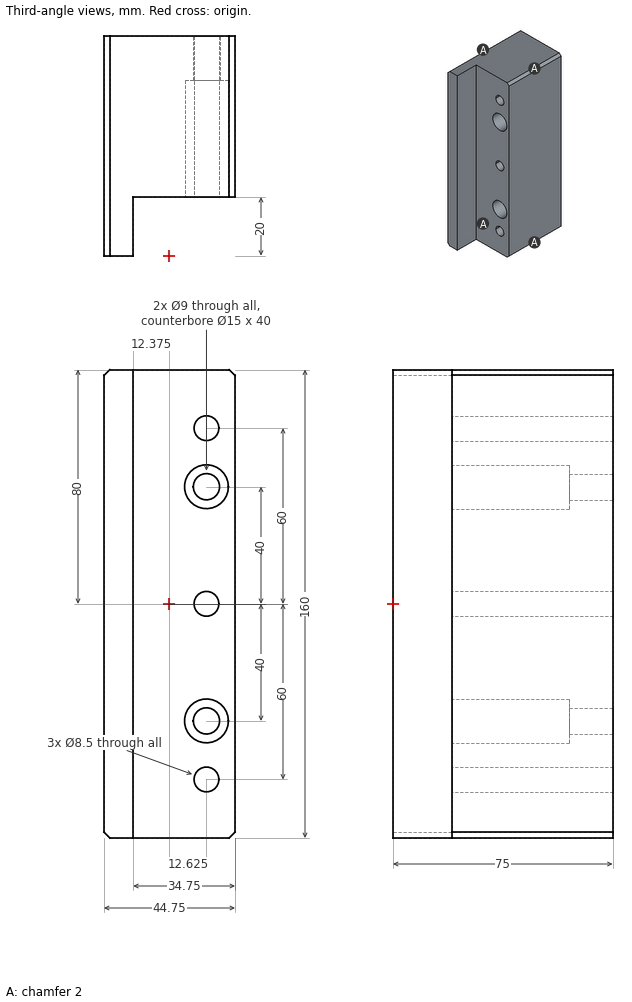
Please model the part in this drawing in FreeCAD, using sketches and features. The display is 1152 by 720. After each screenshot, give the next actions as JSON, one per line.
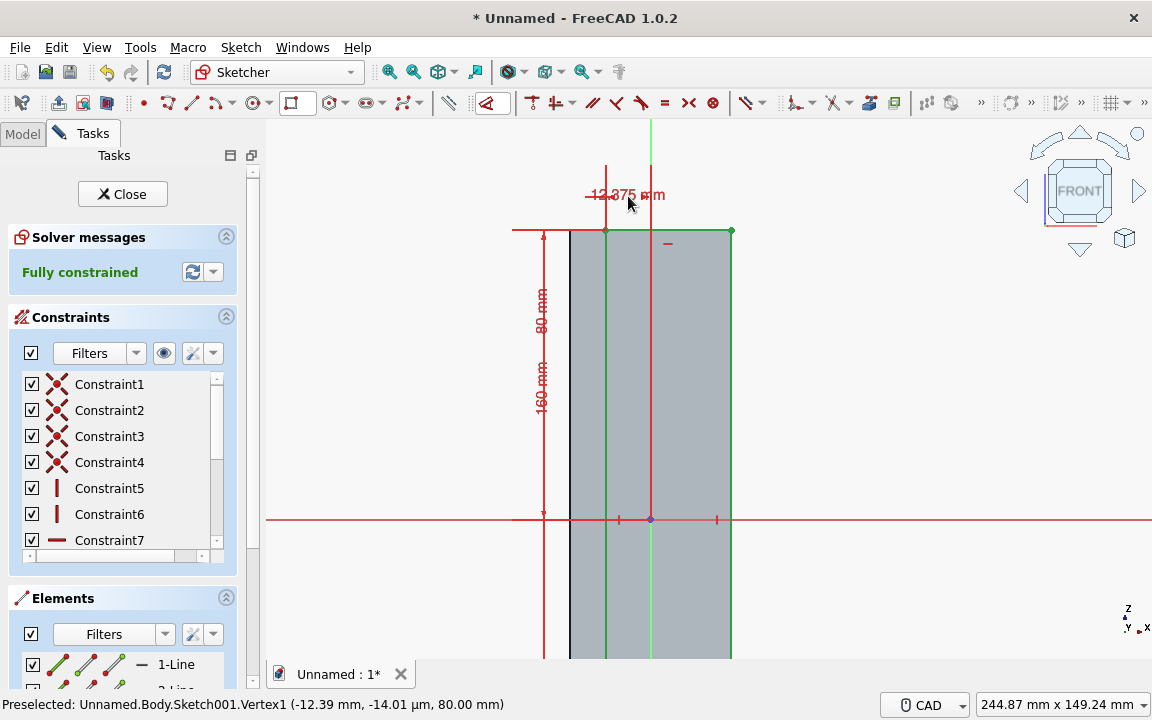
{"action": "left_click", "coordinate": [123, 194]}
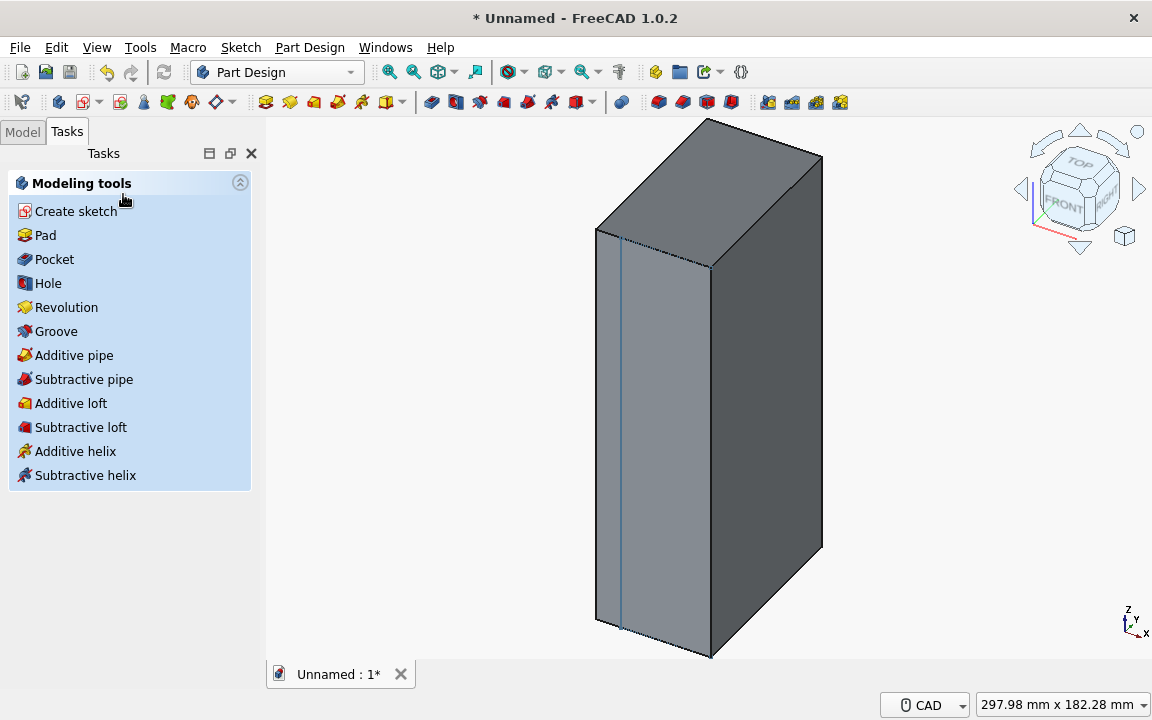
{"action": "left_click", "coordinate": [432, 102]}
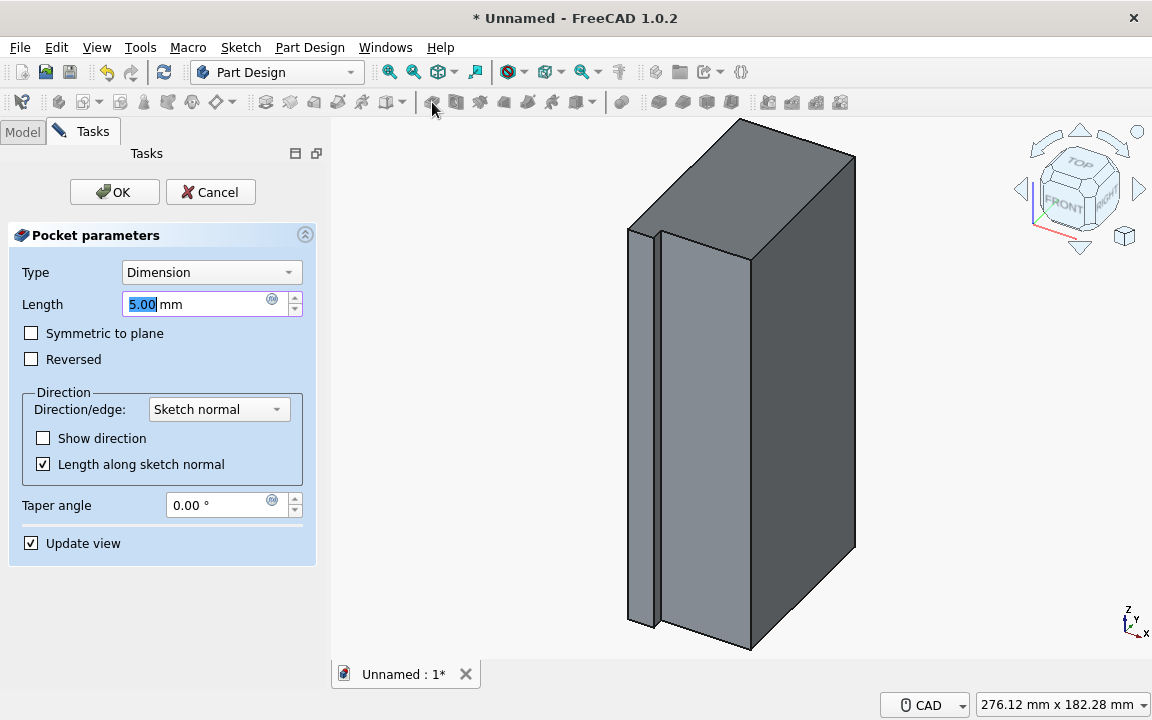
{"action": "type", "text": "20"}
{"action": "key", "text": "Tab"}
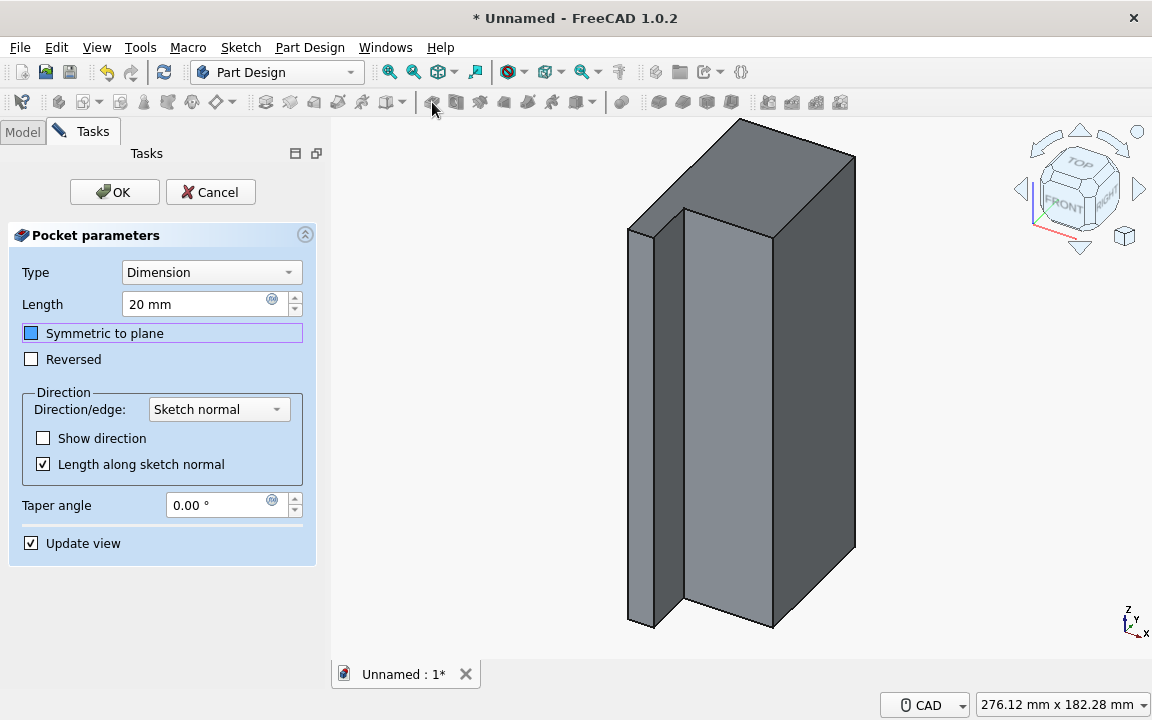
{"action": "left_click", "coordinate": [115, 192]}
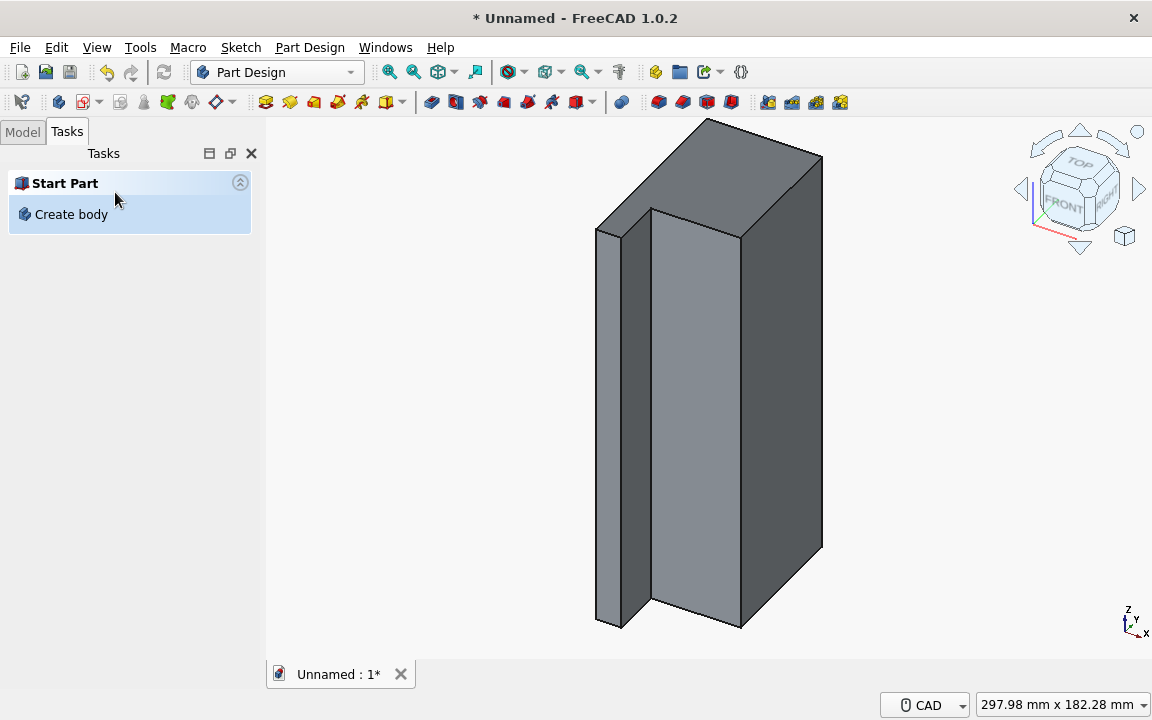
{"action": "key", "text": "4"}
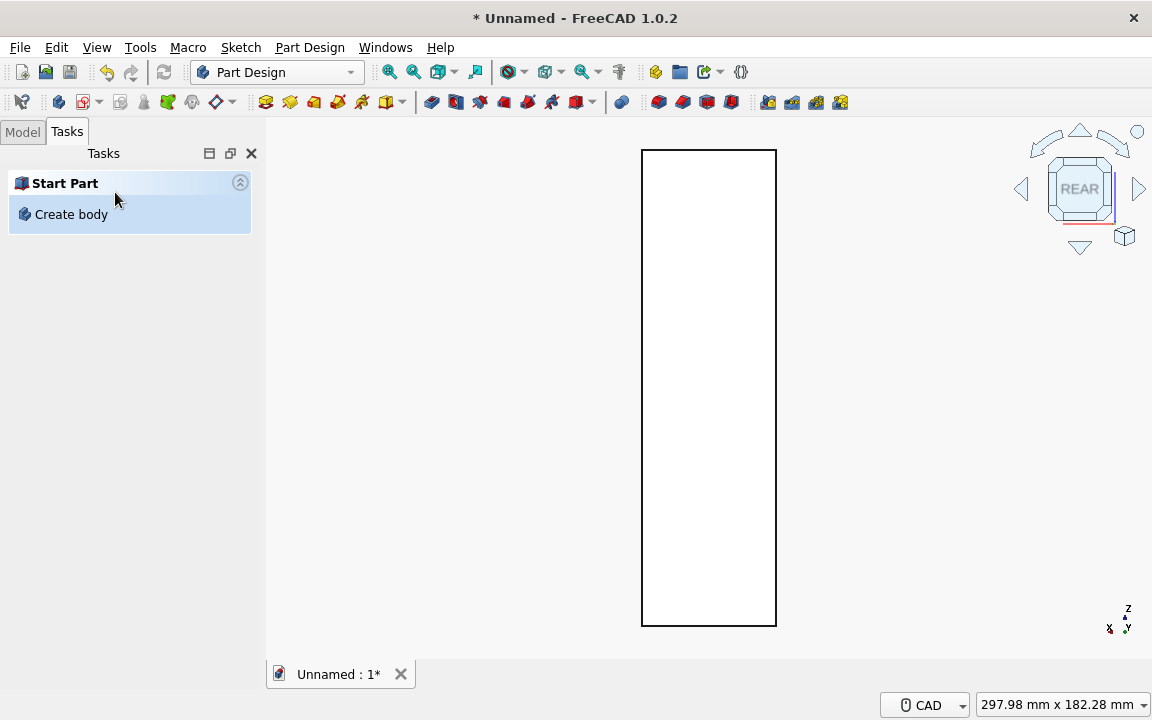
{"action": "left_click", "coordinate": [709, 251]}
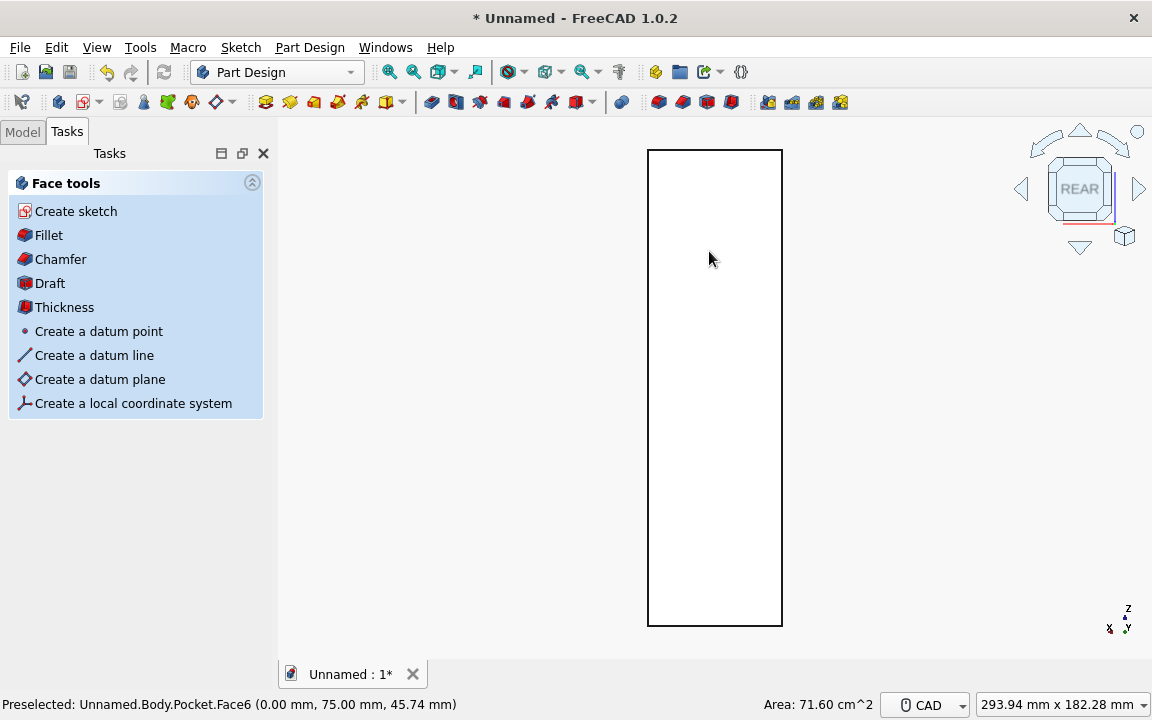
{"action": "left_click", "coordinate": [84, 102]}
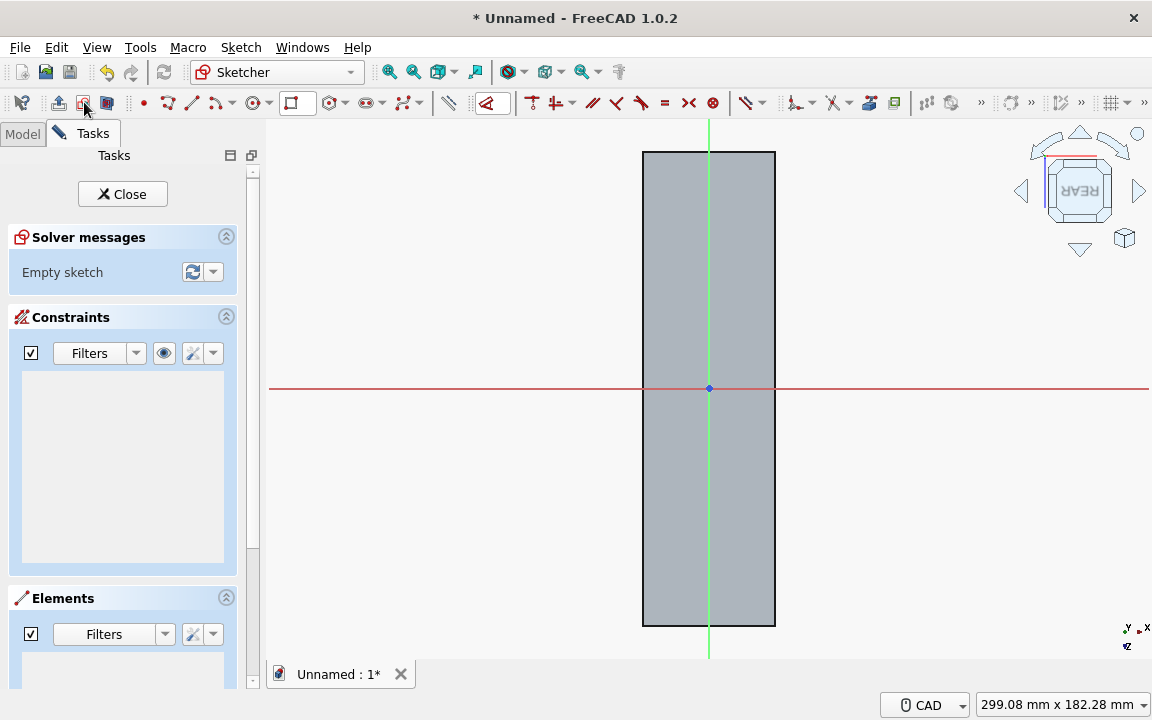
{"action": "left_click", "coordinate": [254, 104]}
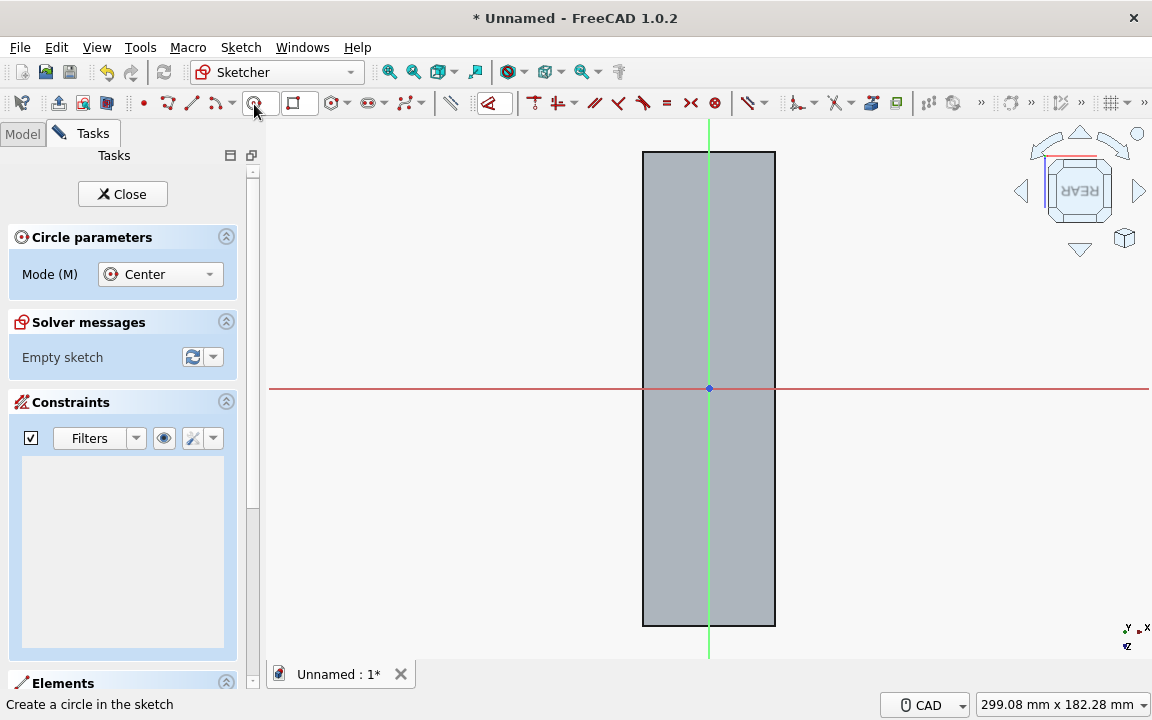
{"action": "scroll", "coordinate": [746, 211], "scroll_direction": "up", "scroll_amount": 3}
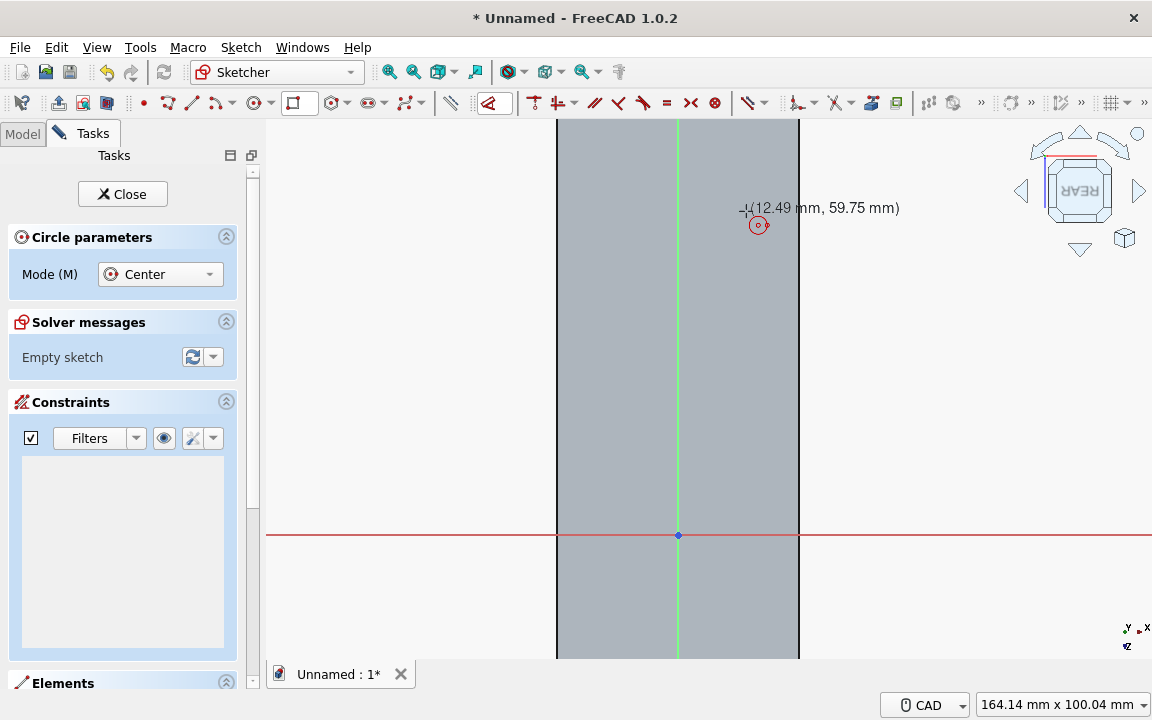
{"action": "left_click", "coordinate": [746, 211]}
{"action": "left_click", "coordinate": [763, 195]}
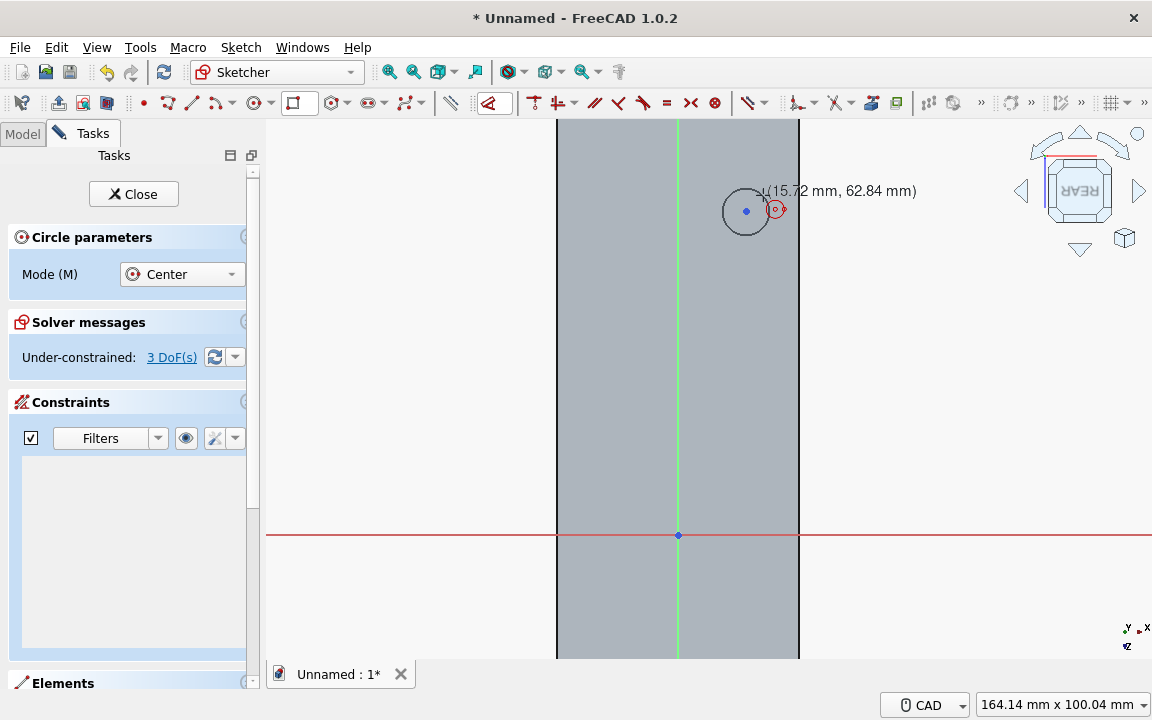
{"action": "left_click", "coordinate": [746, 535]}
{"action": "left_click", "coordinate": [763, 519]}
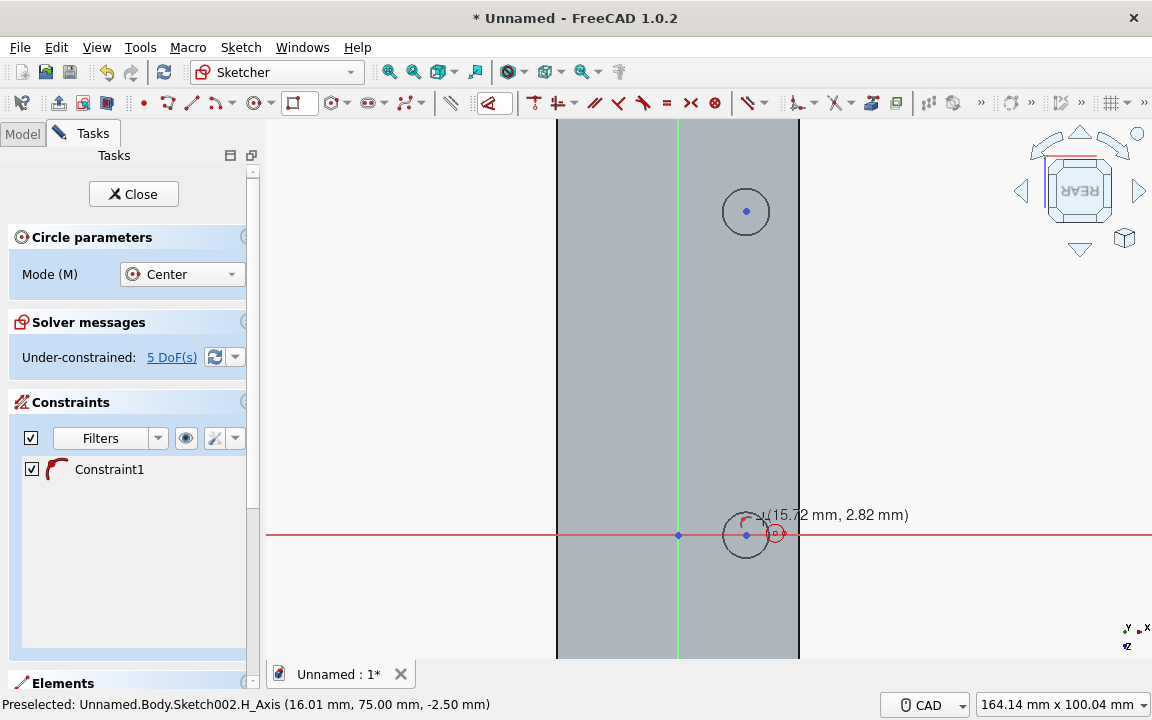
{"action": "scroll", "coordinate": [573, 270], "scroll_direction": "down", "scroll_amount": 4}